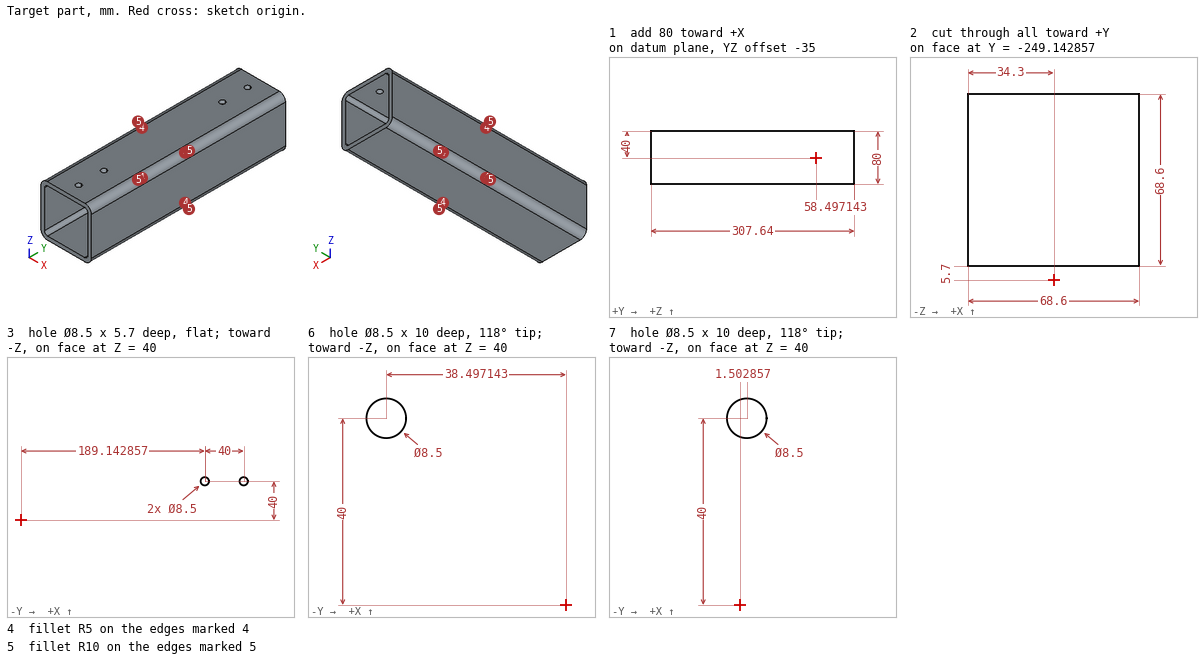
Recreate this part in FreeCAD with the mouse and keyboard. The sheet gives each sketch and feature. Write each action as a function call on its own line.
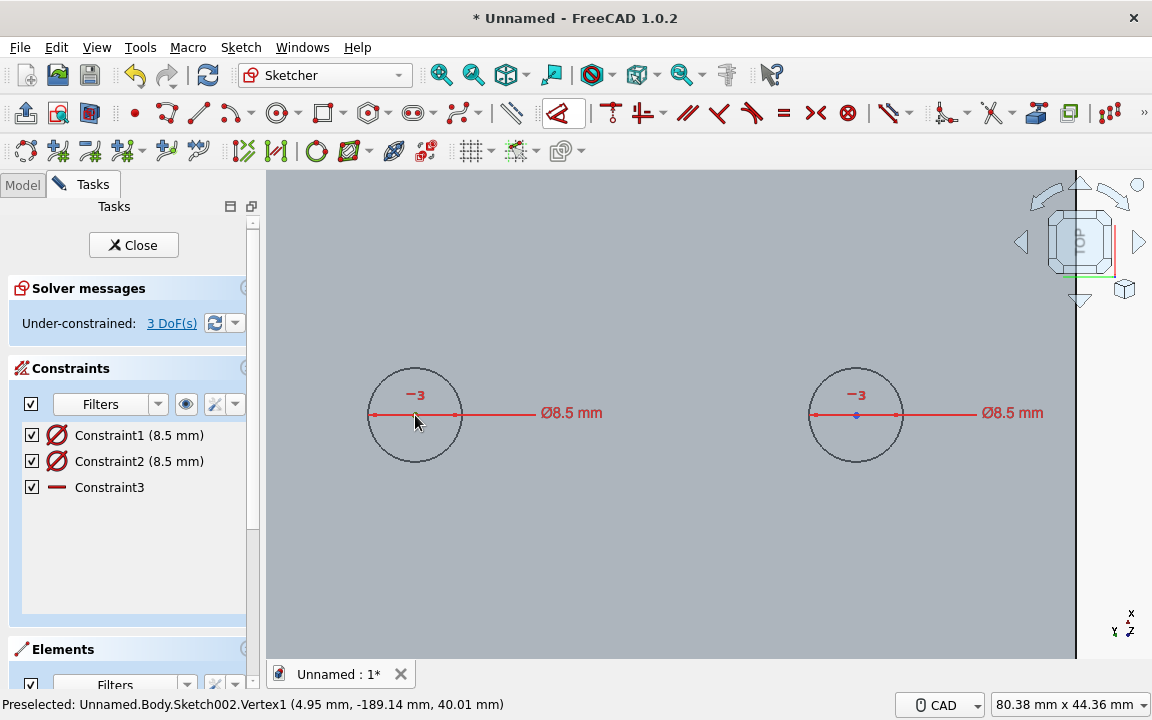
key(i)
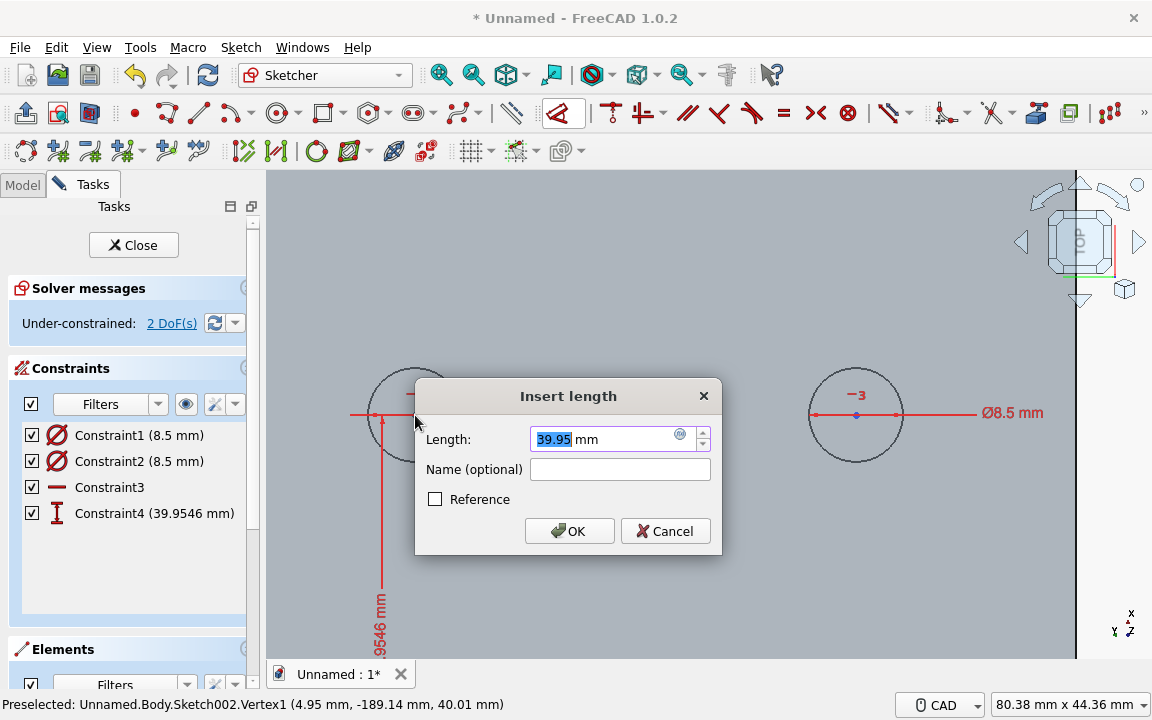
text(40)
key(Return)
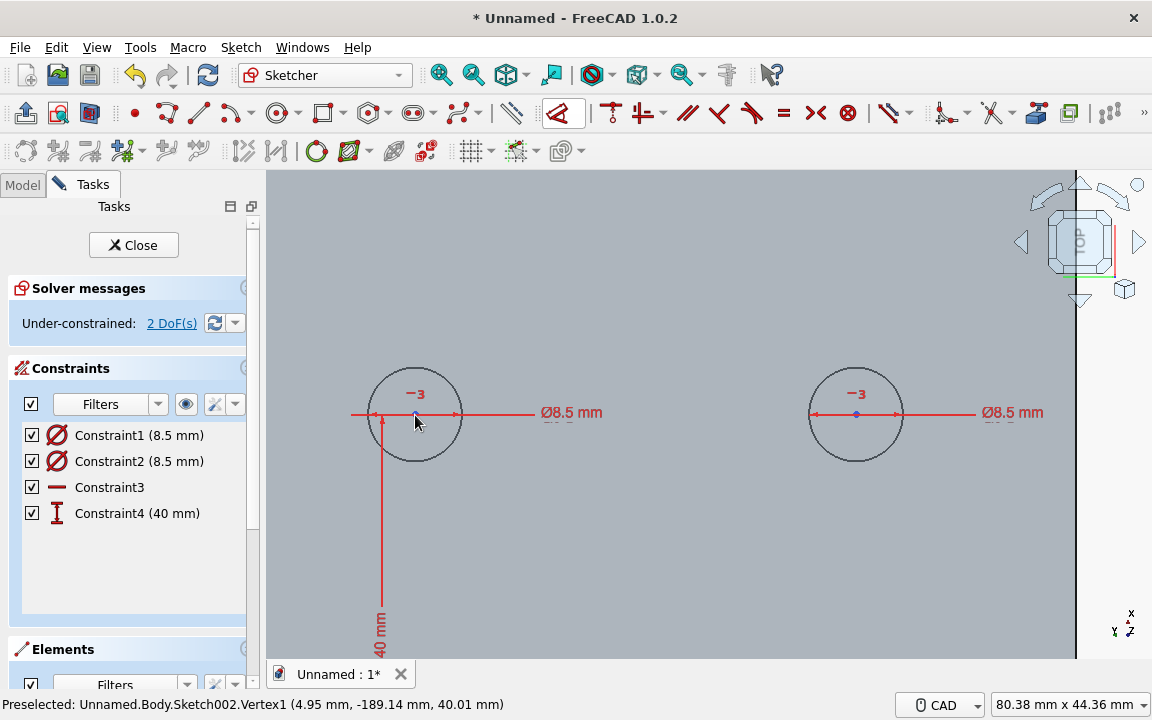
click(415, 414)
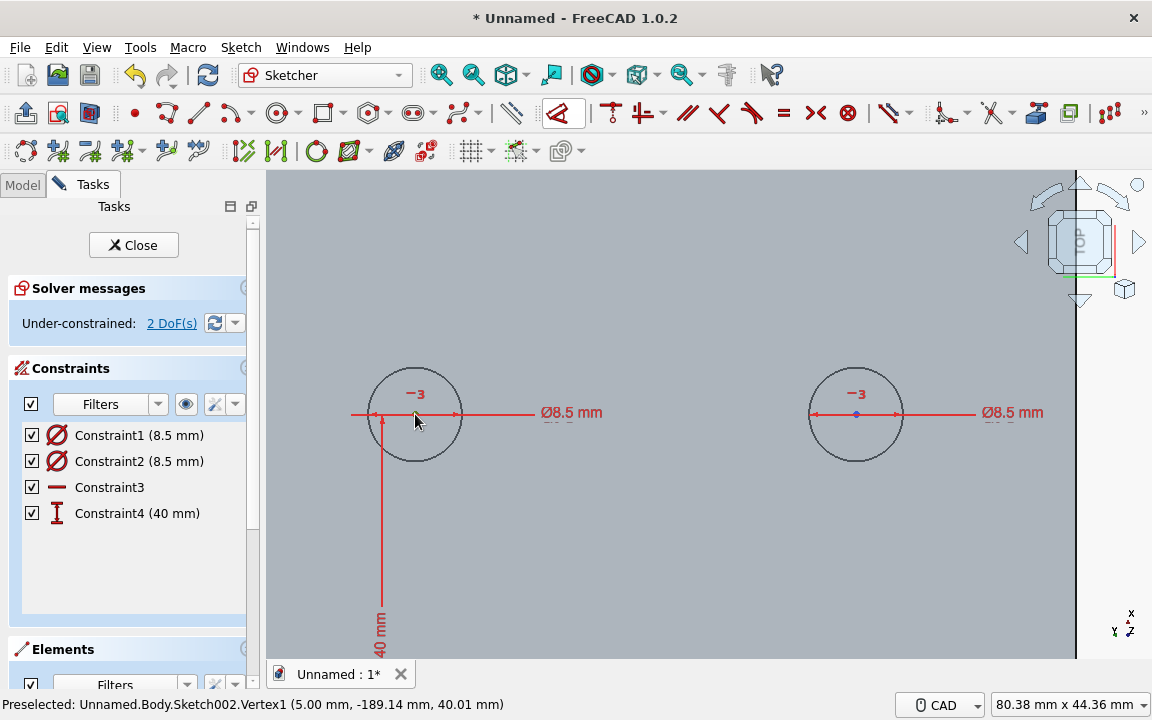
click(856, 414)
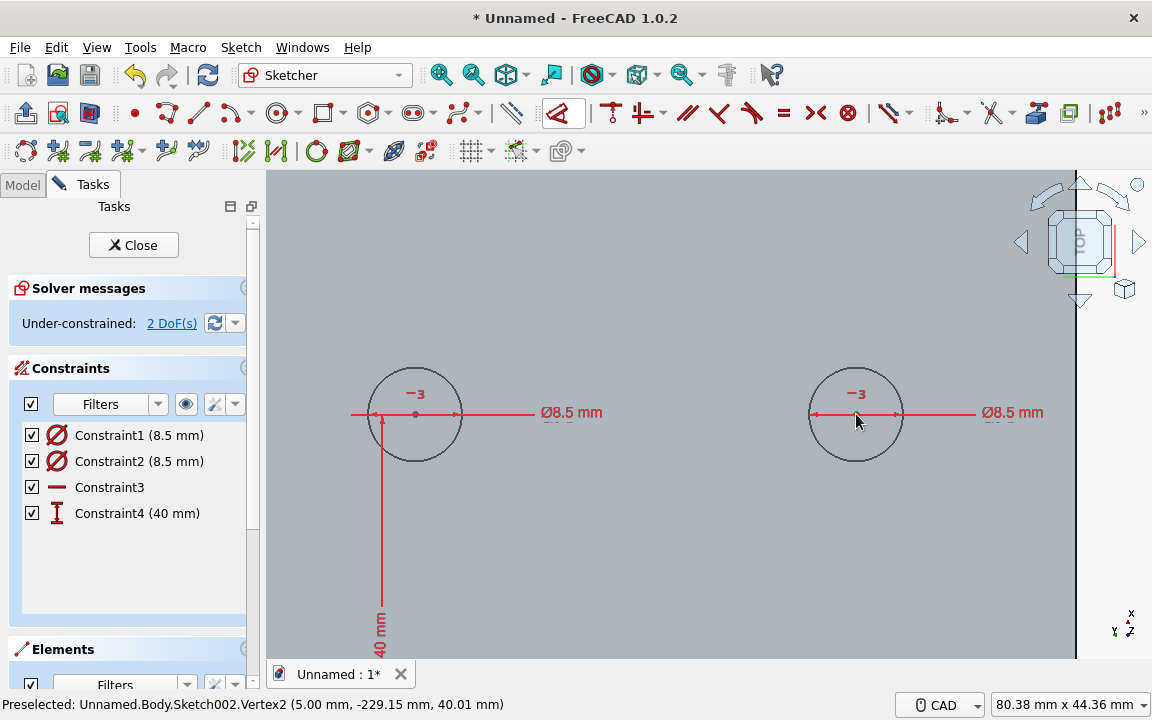
click(580, 114)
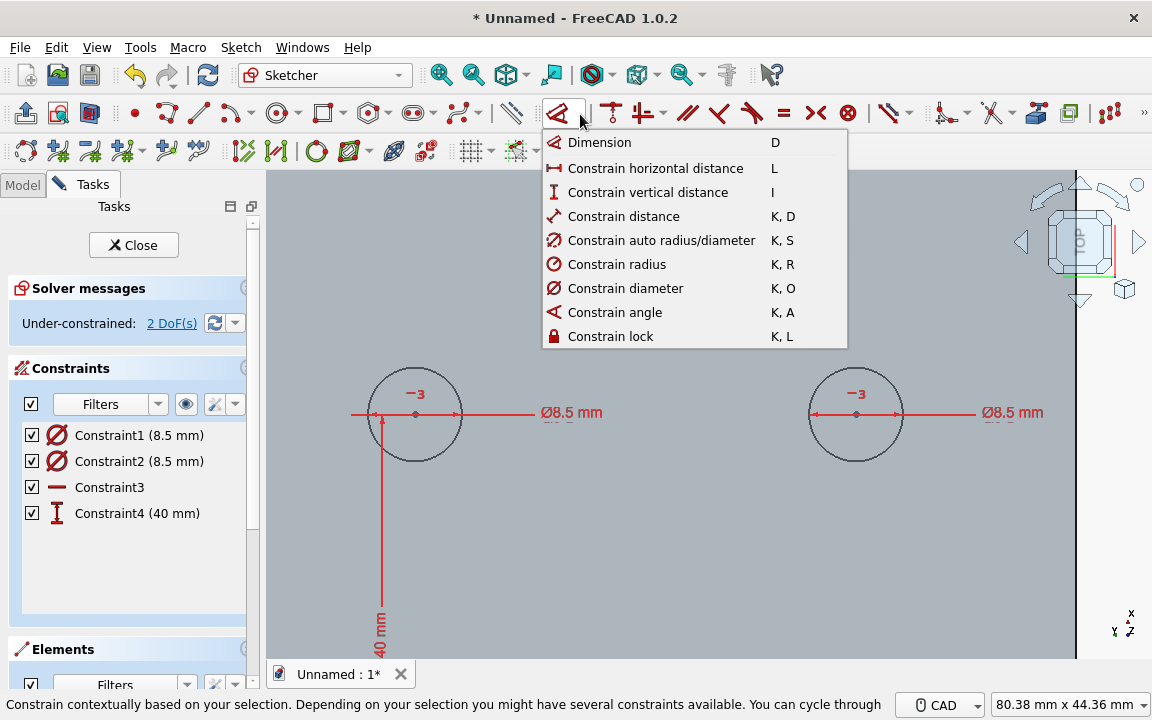
click(695, 168)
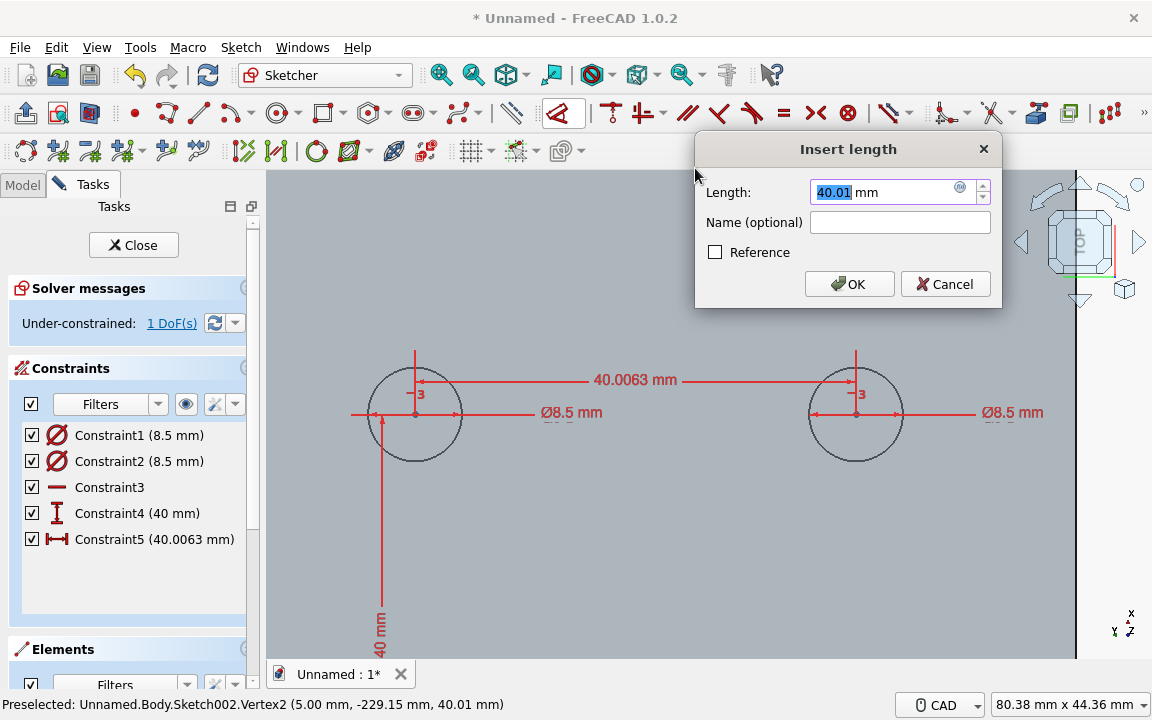
text(40)
key(Return)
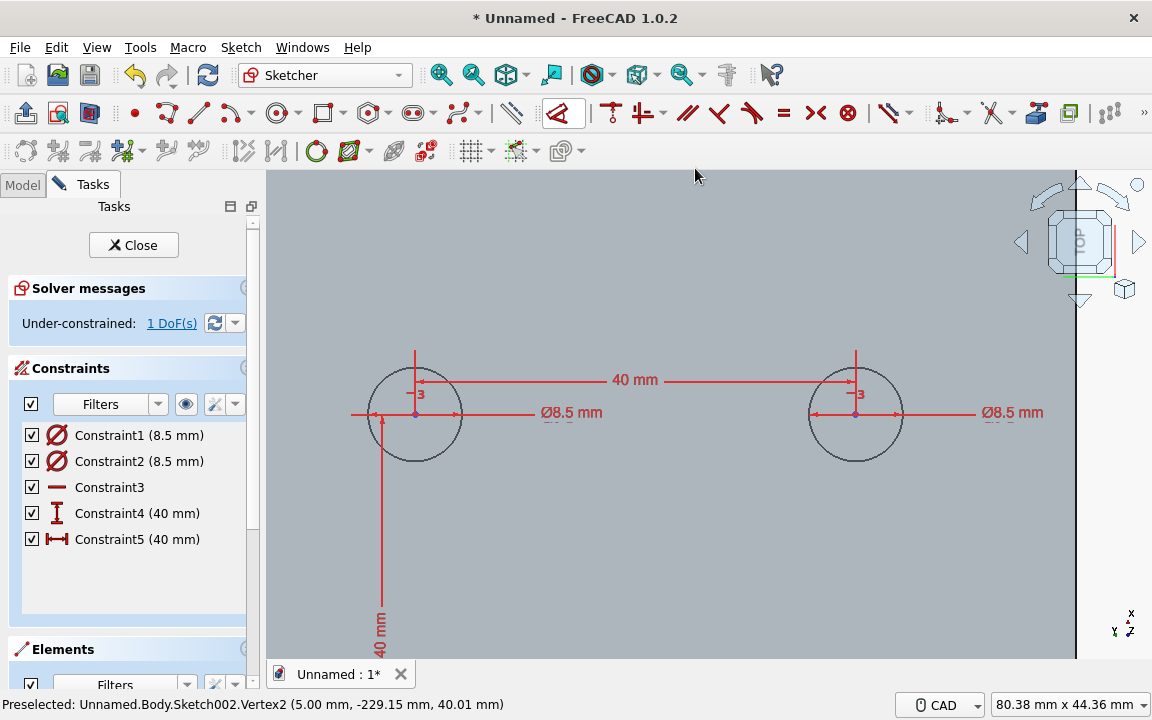
click(415, 414)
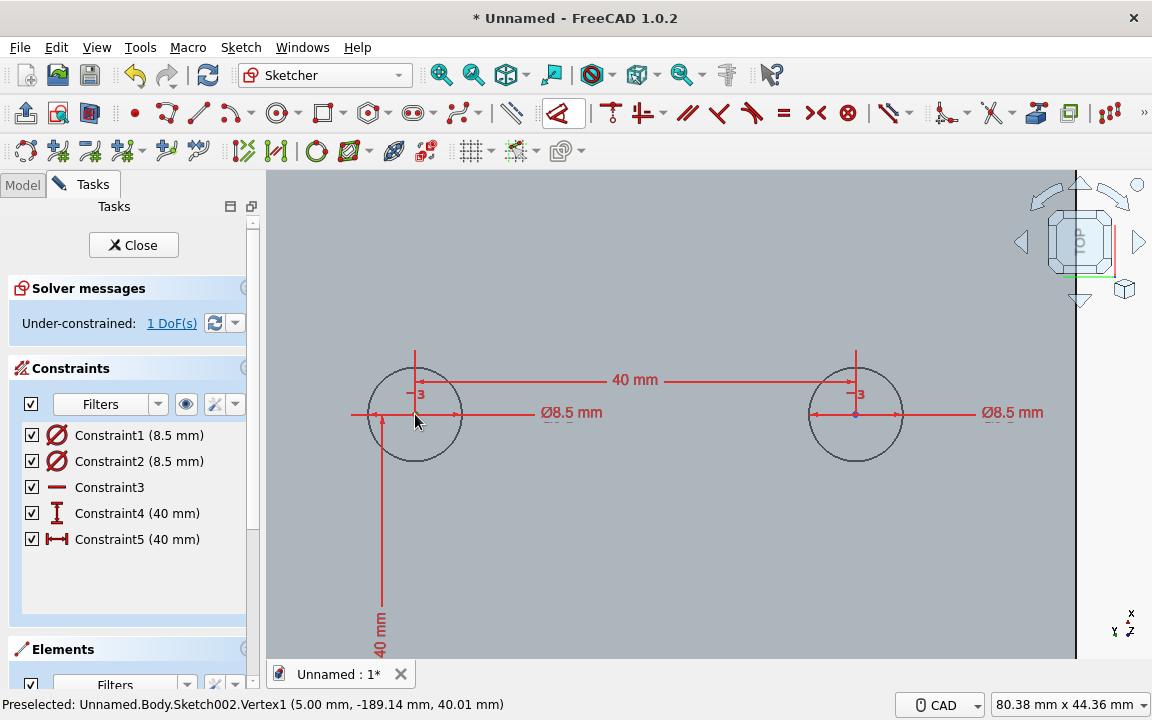
key(l)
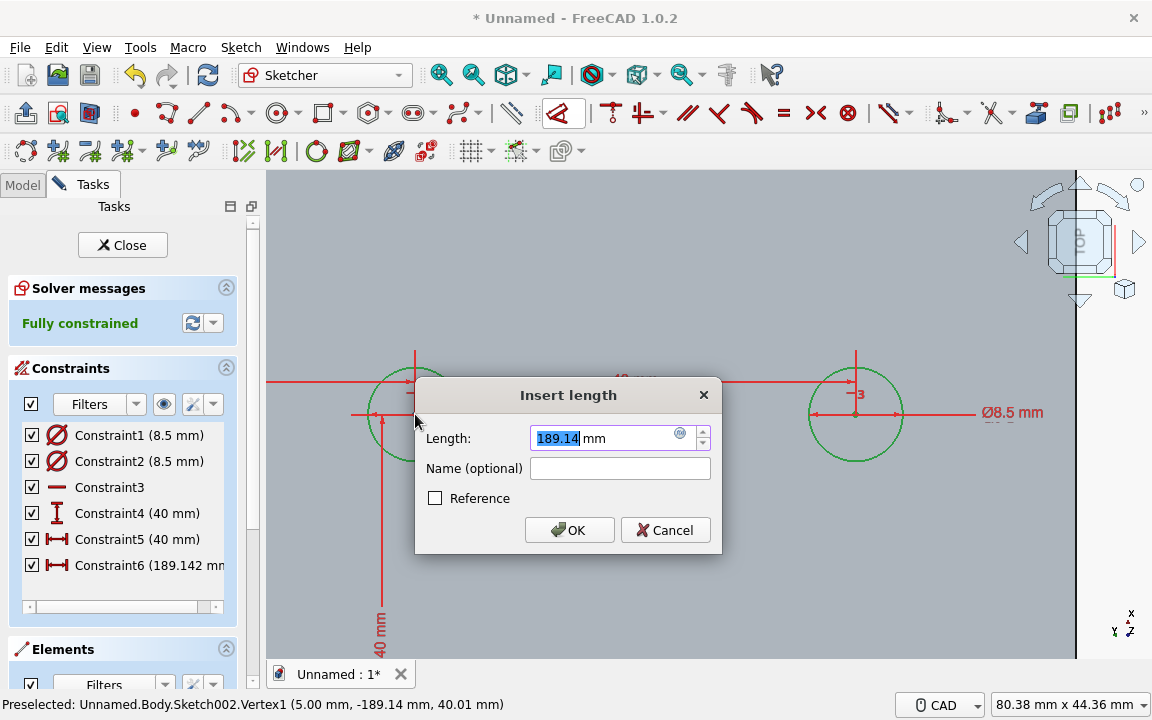
text(189.142857)
key(Return)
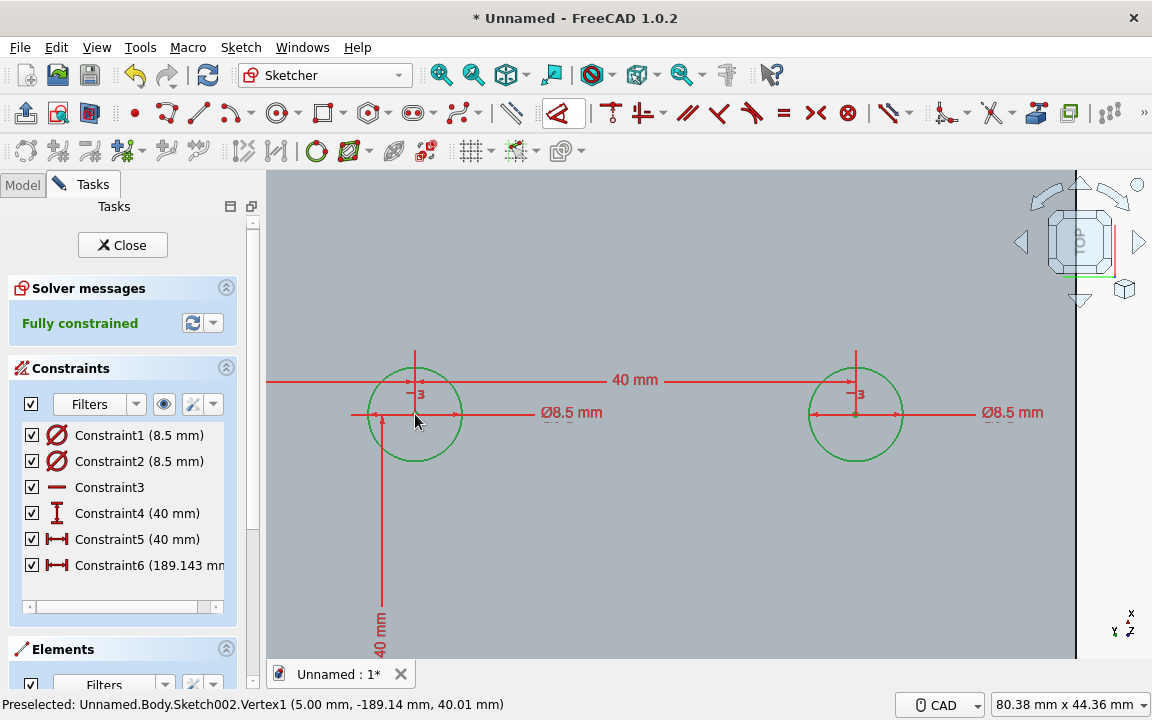
click(123, 245)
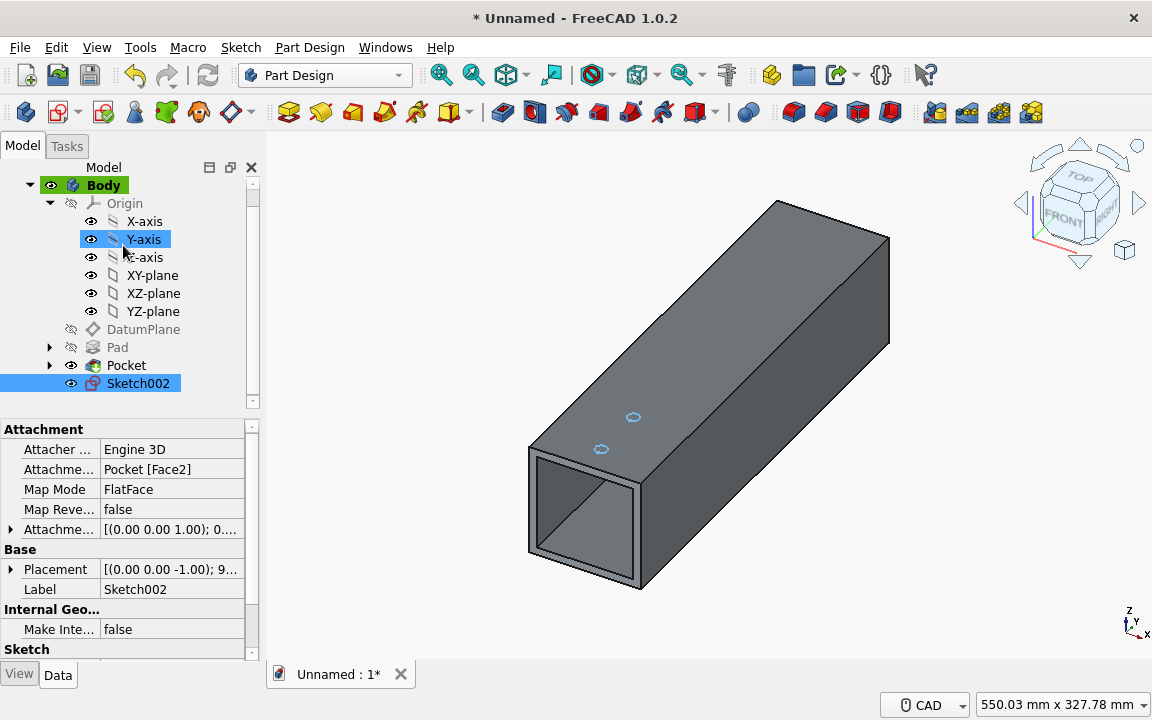
click(536, 112)